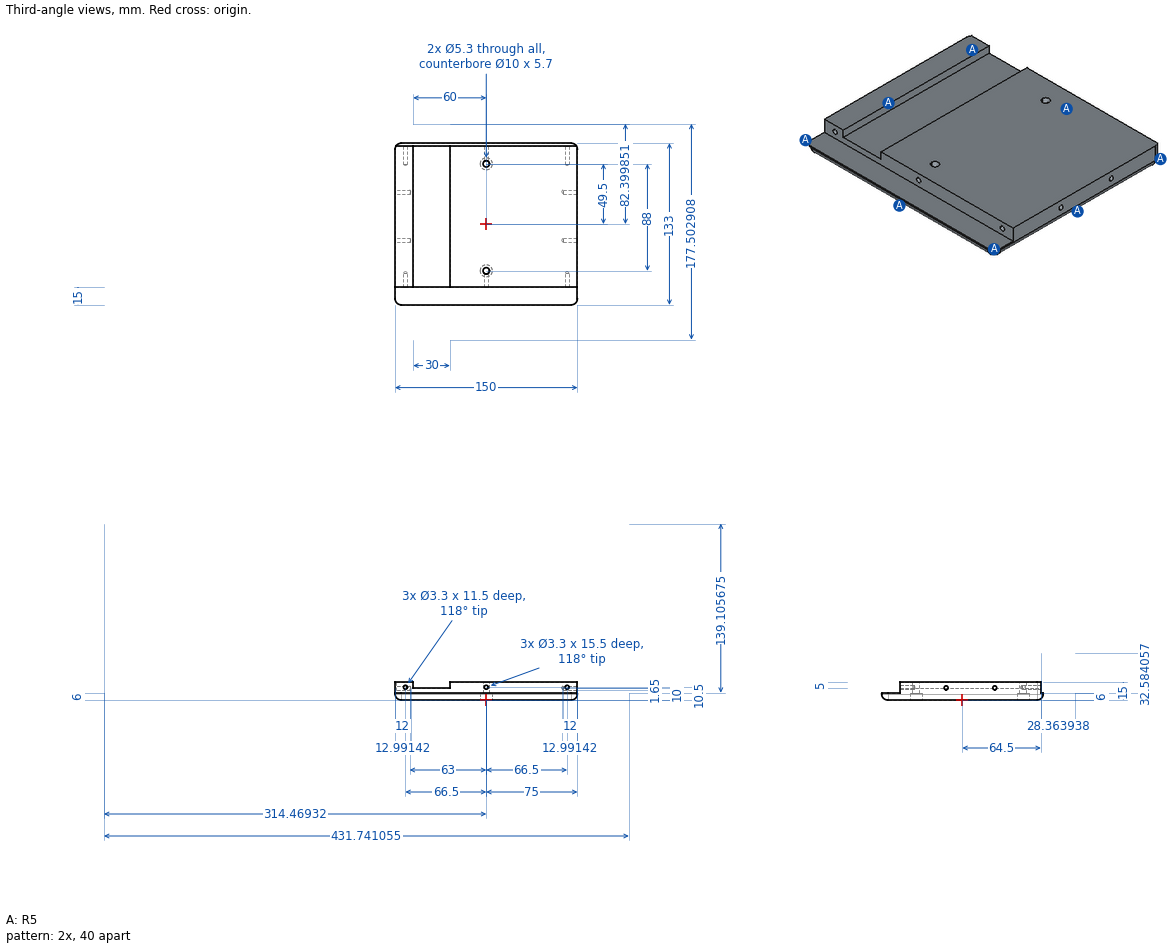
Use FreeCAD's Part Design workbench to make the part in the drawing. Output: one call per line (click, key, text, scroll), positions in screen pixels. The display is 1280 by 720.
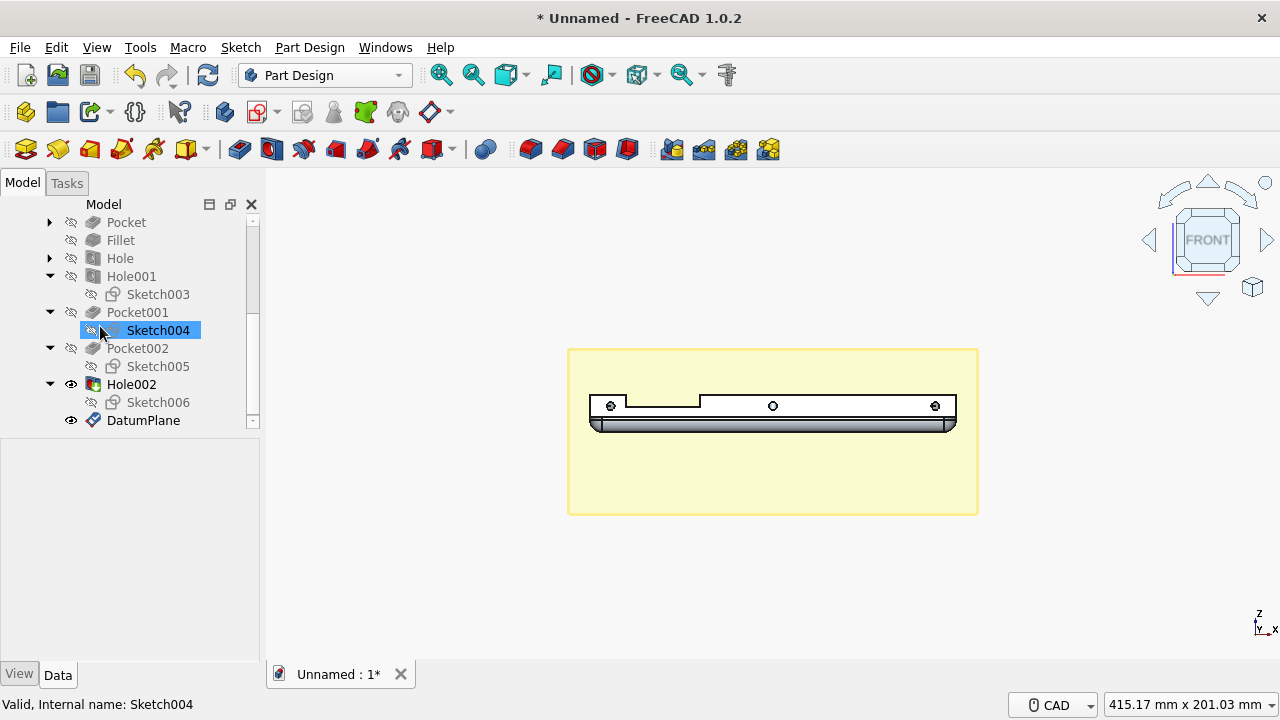
click(116, 420)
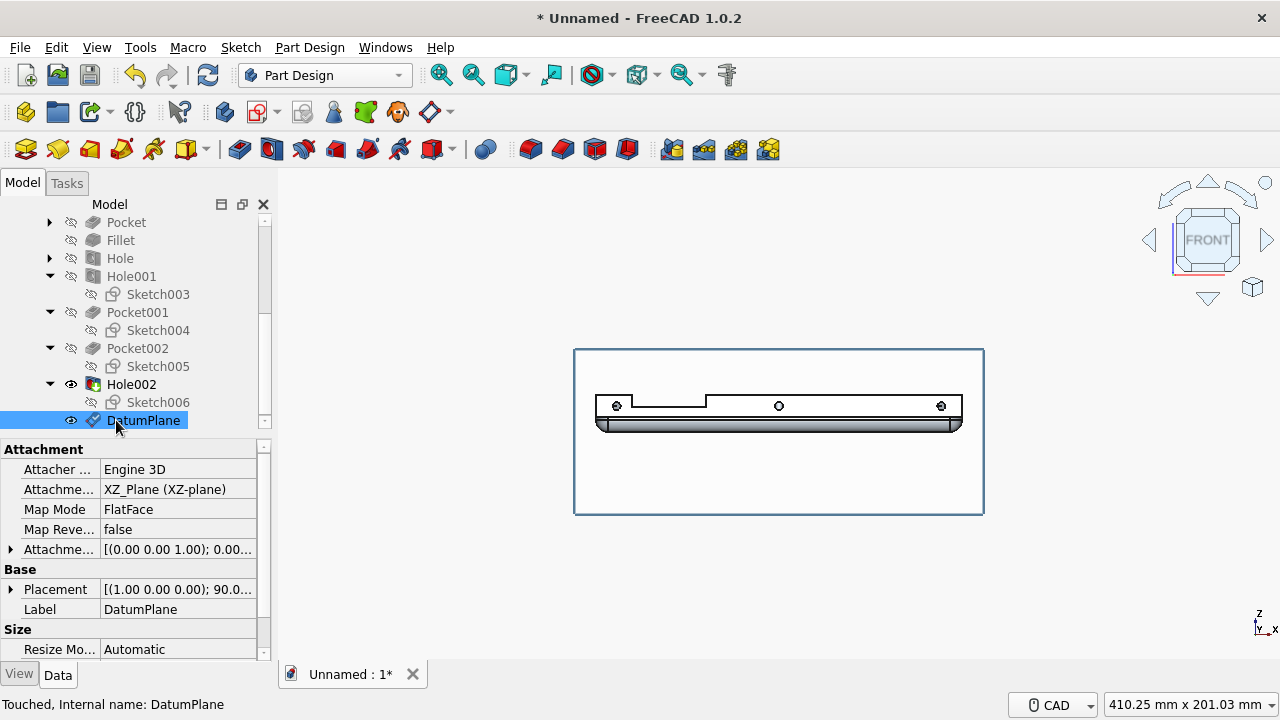
click(258, 112)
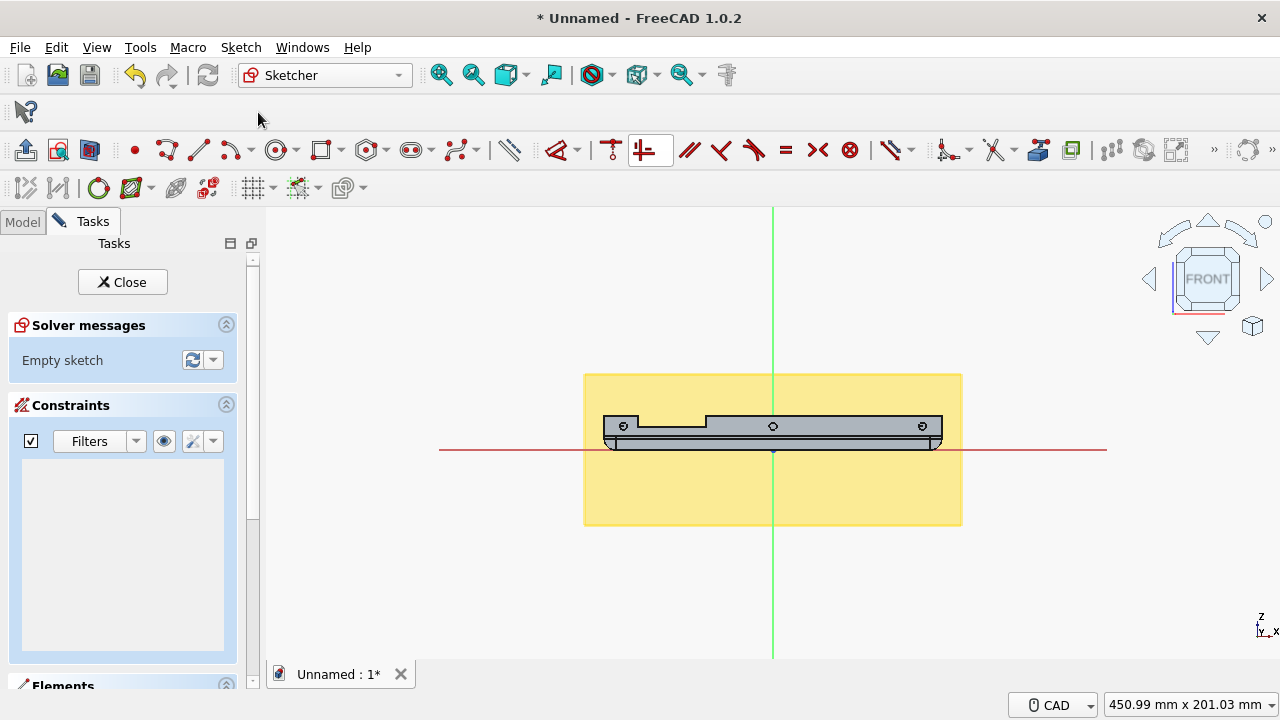
click(90, 150)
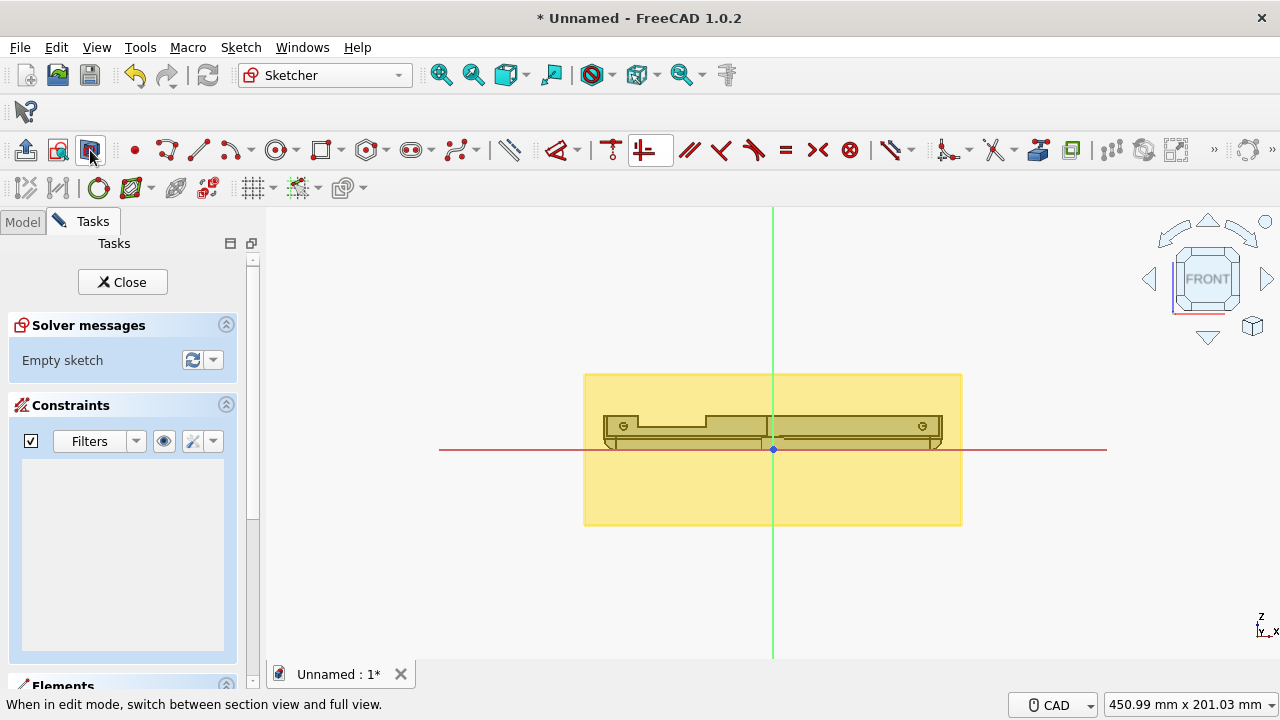
scroll(939, 429, up, 13)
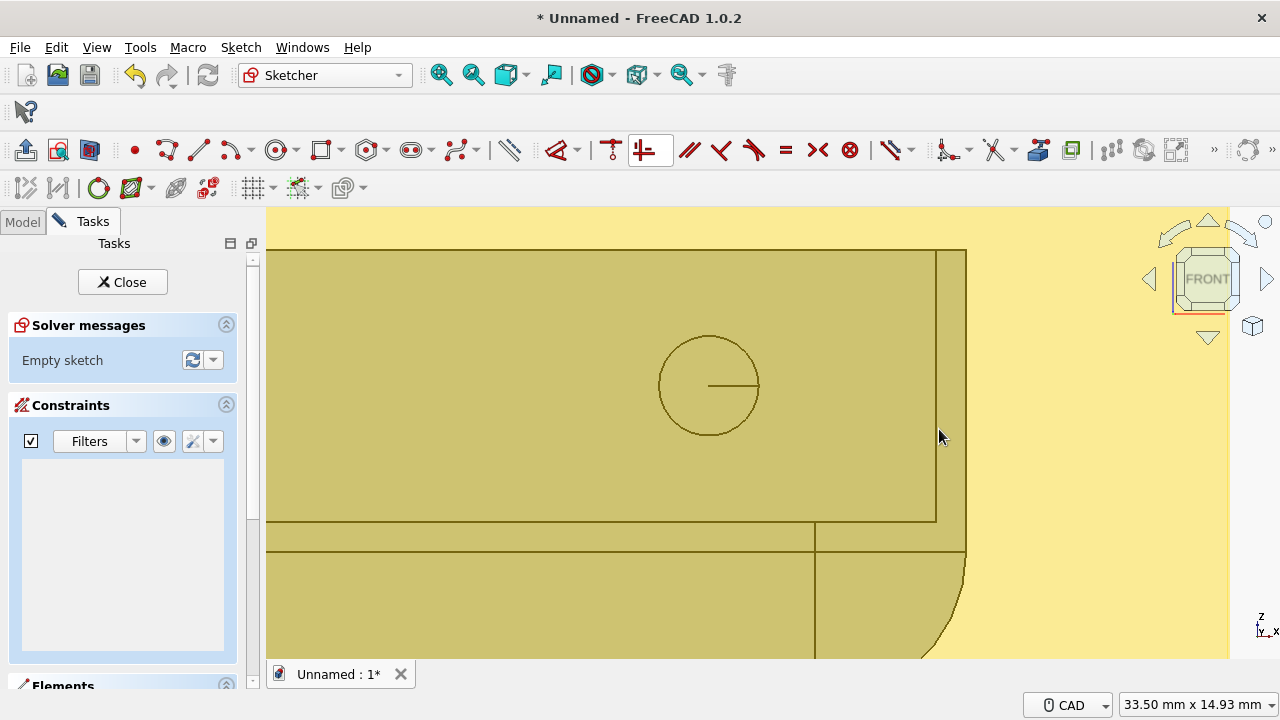
click(168, 150)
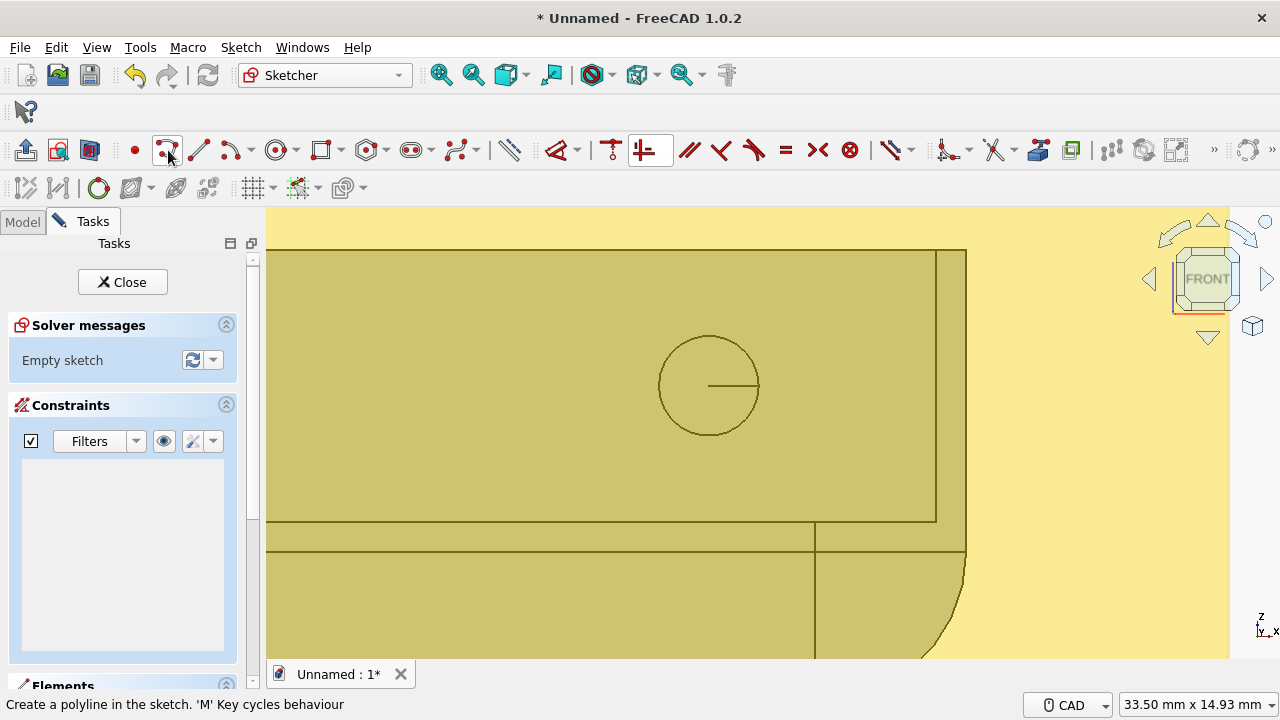
click(573, 401)
click(966, 401)
click(966, 451)
click(603, 451)
click(573, 402)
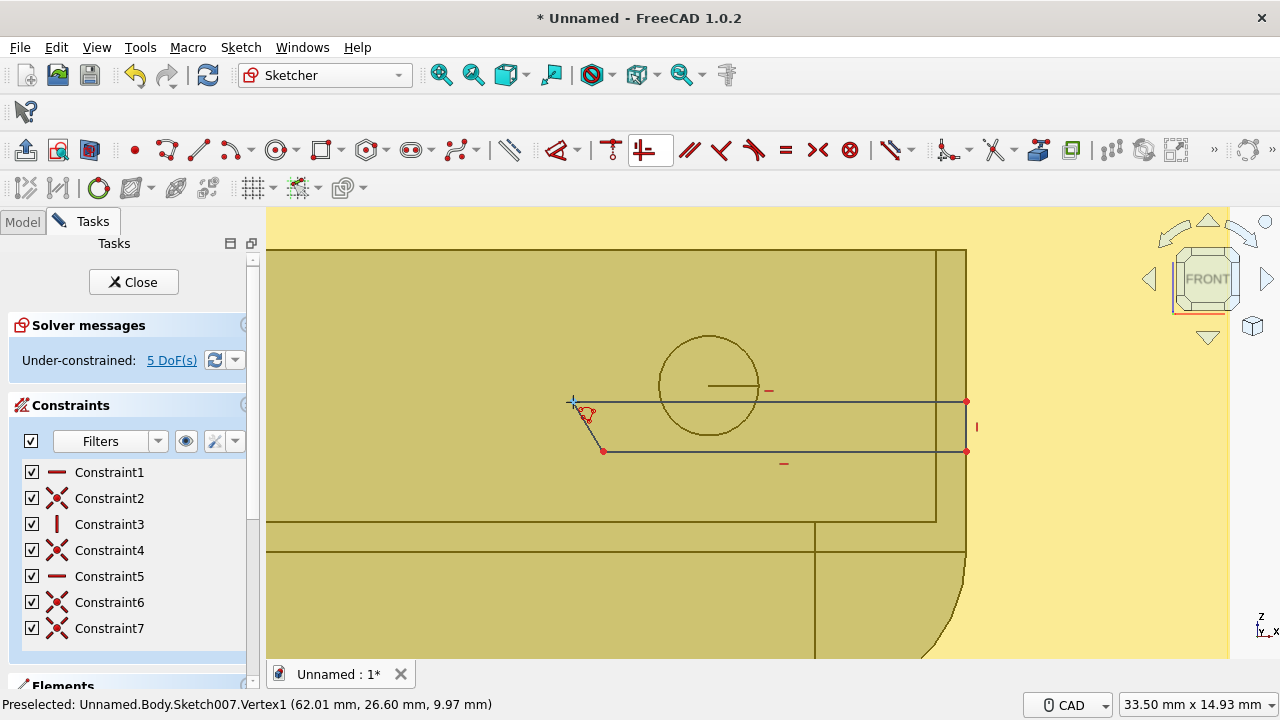
click(200, 150)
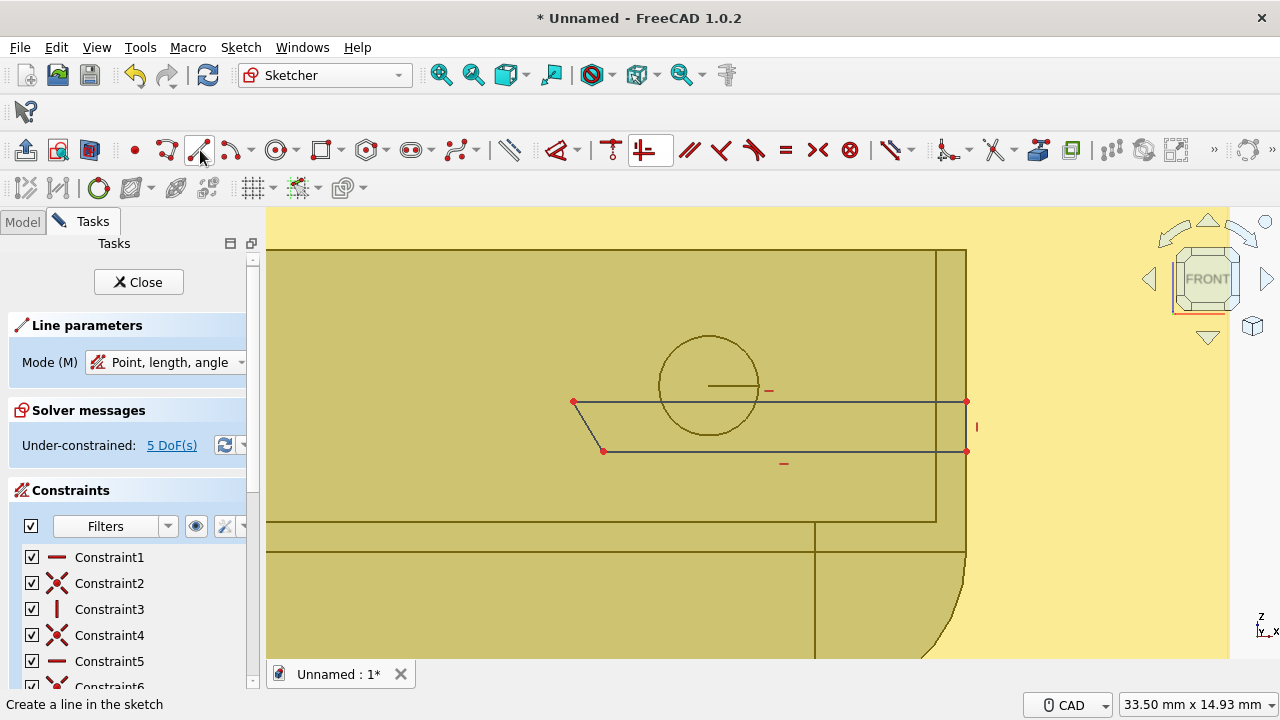
click(534, 401)
click(416, 401)
key(Escape)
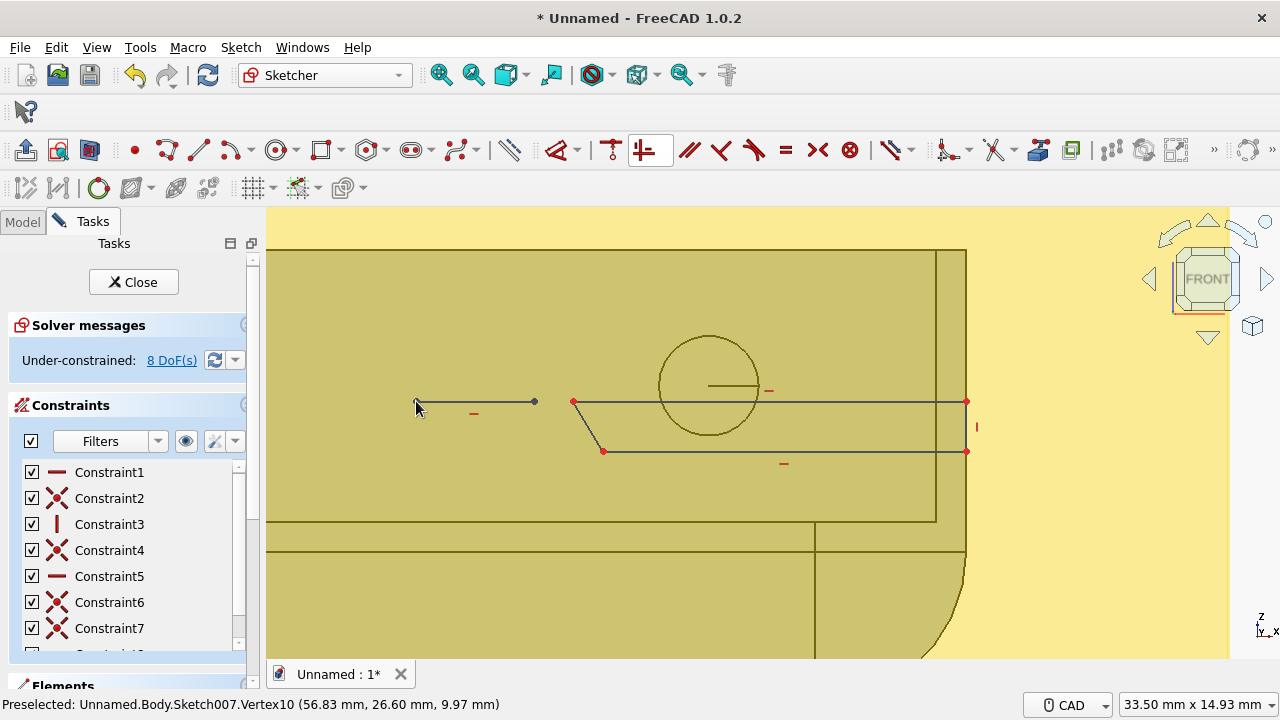
click(499, 402)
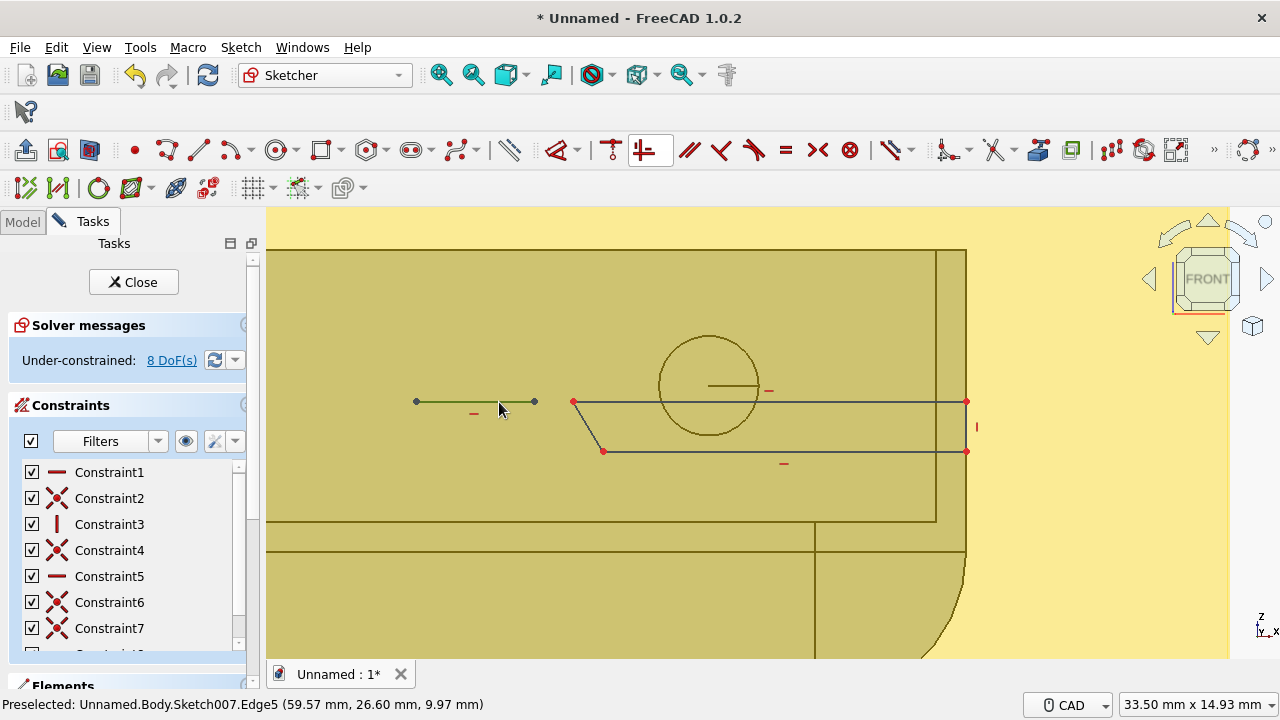
click(510, 150)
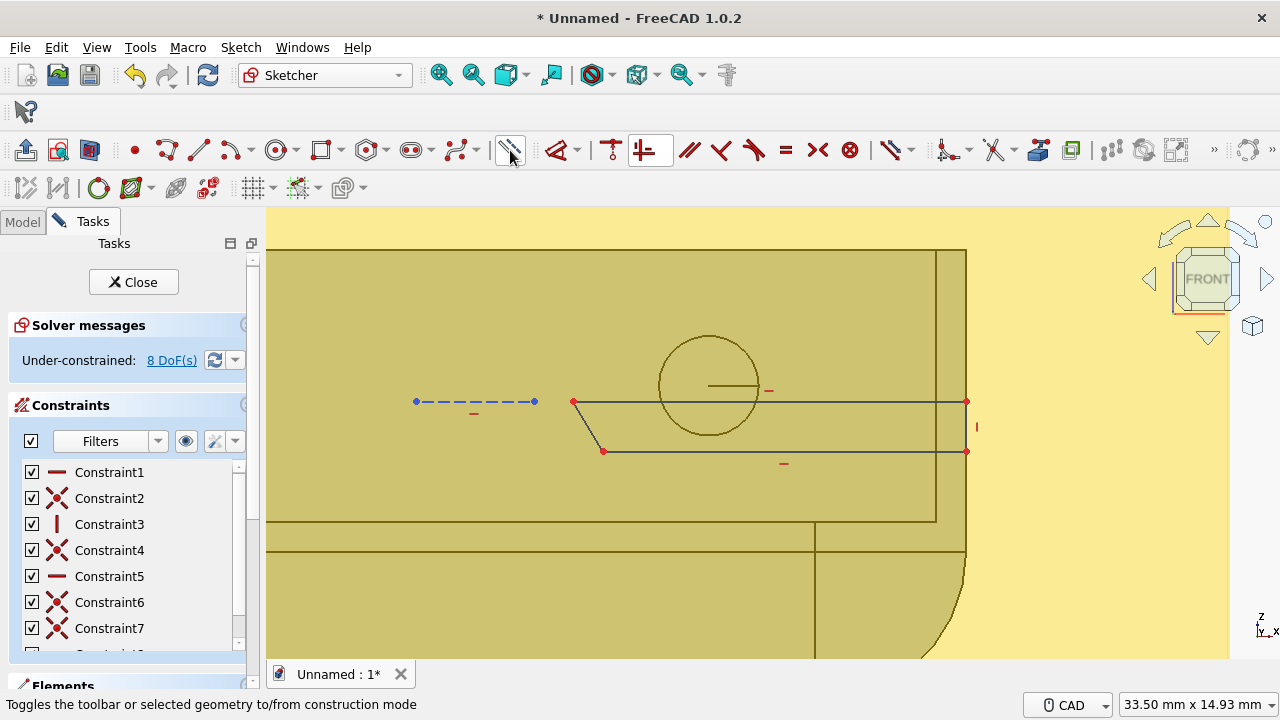
click(556, 150)